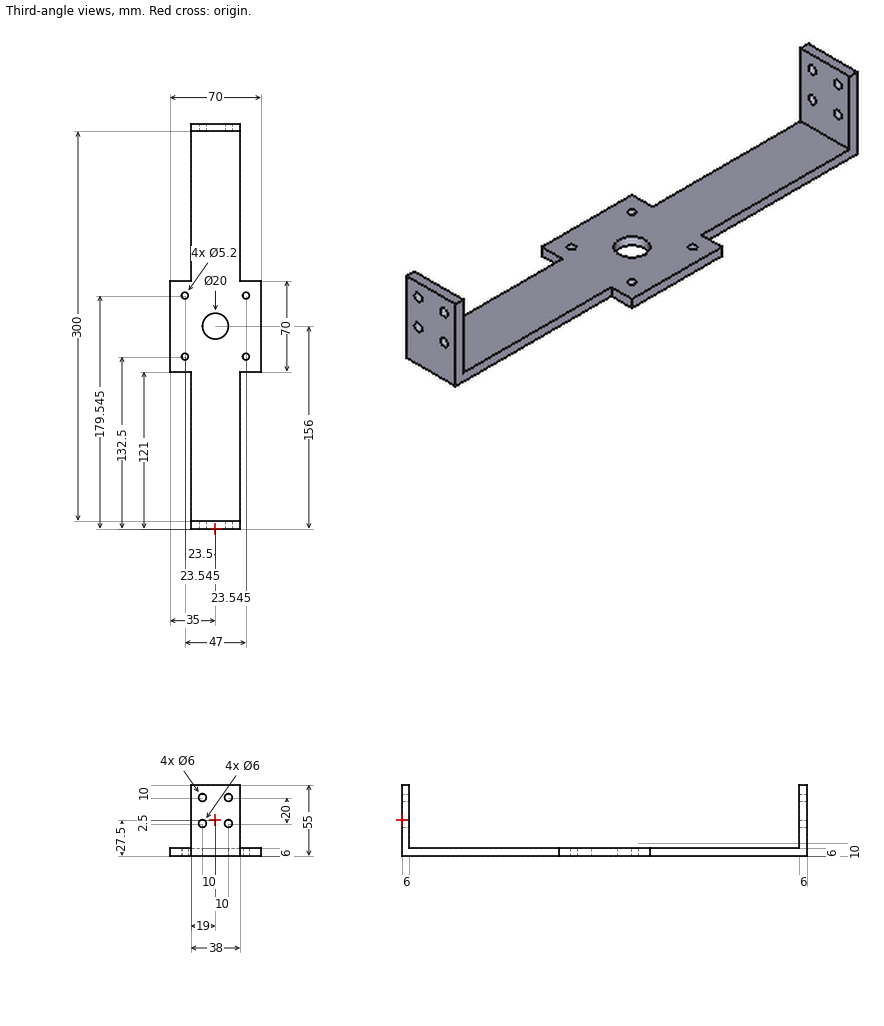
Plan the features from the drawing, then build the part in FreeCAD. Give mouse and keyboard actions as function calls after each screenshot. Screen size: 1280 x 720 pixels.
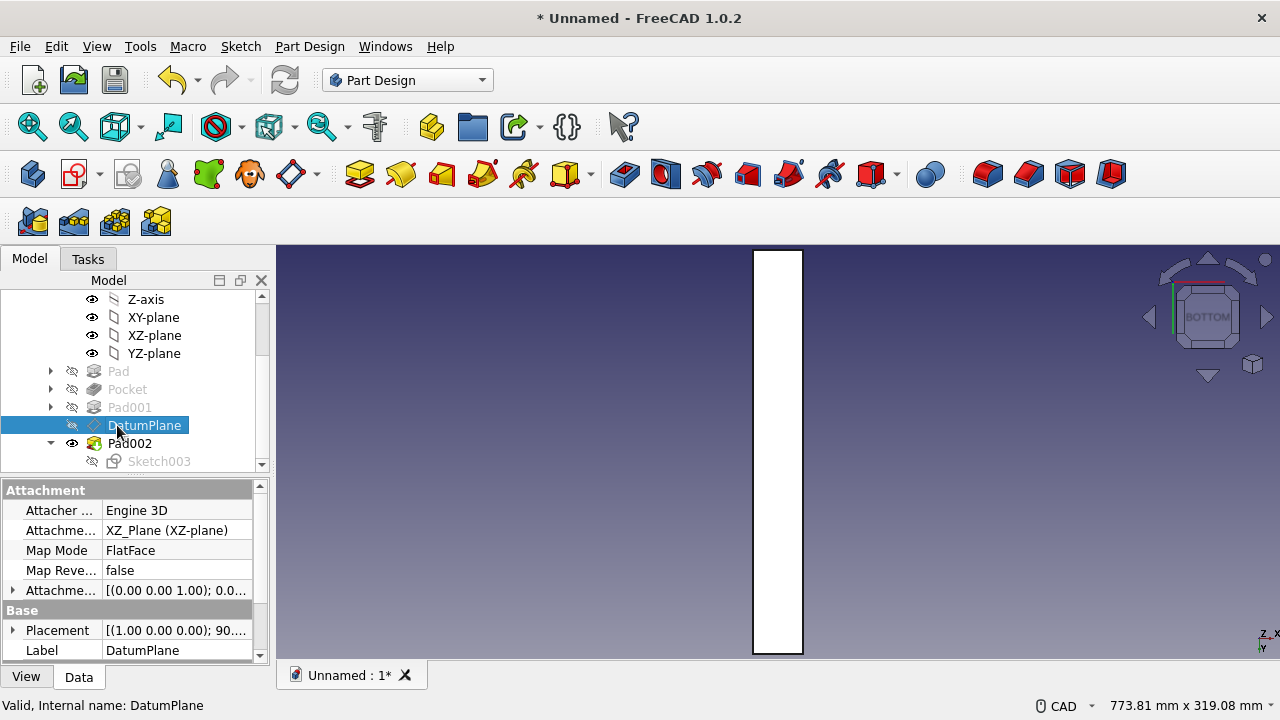
click(778, 624)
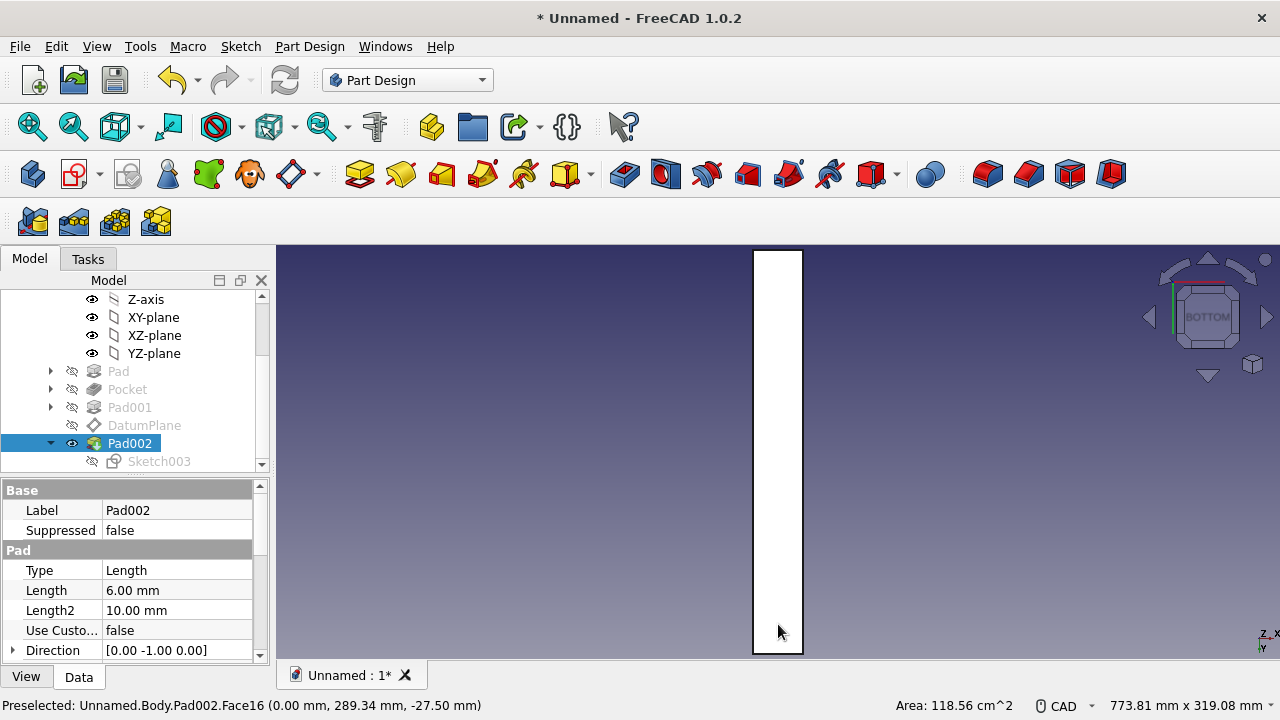
click(74, 174)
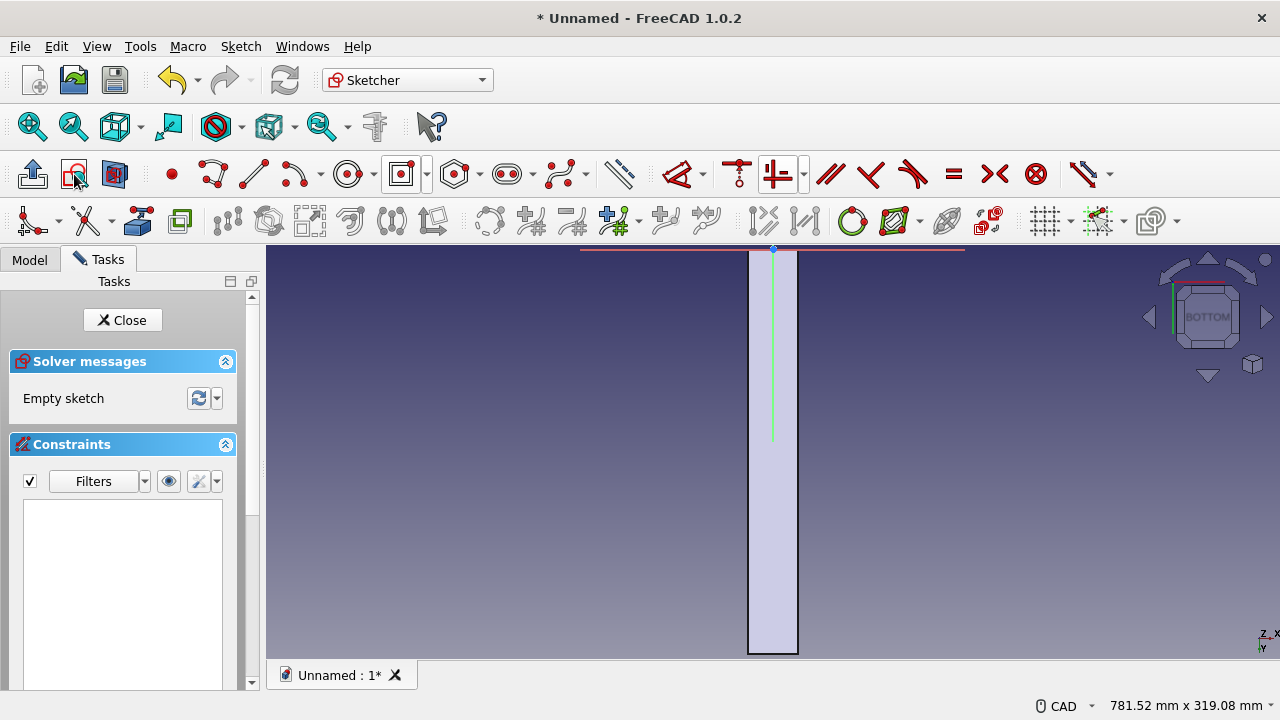
scroll(813, 452, up, 5)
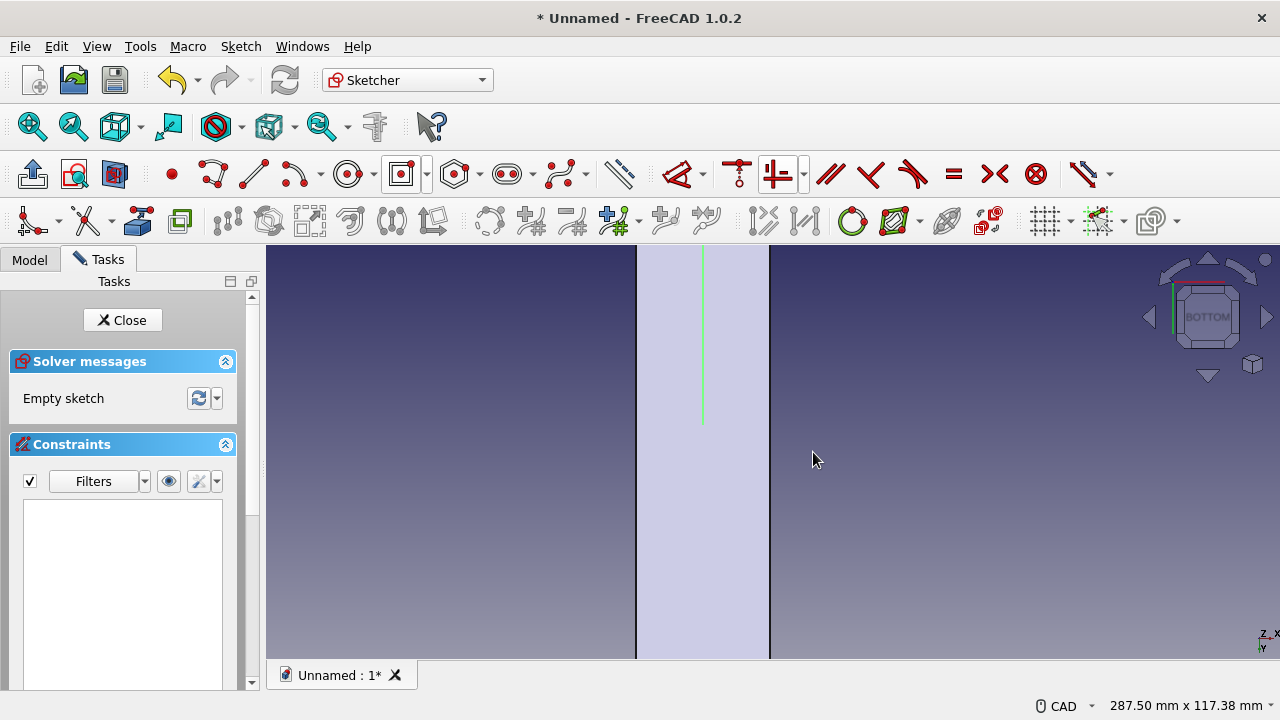
key(g)
key(r)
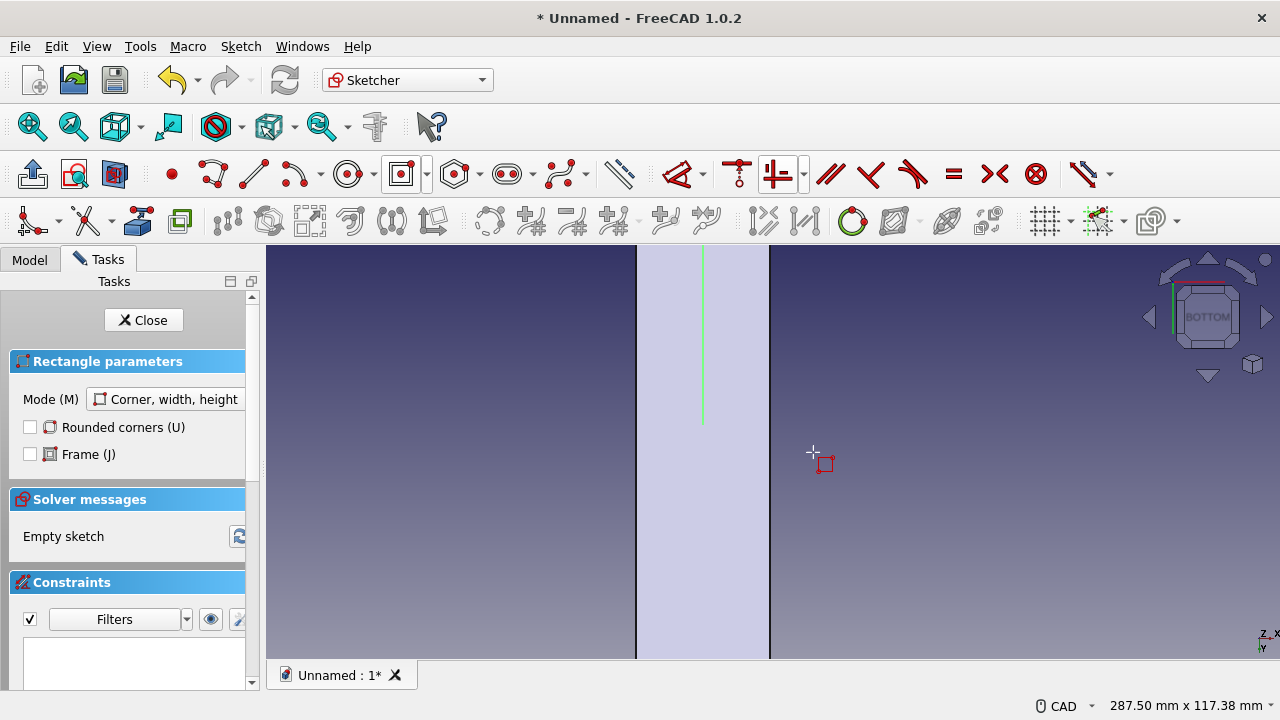
click(580, 328)
move(827, 575)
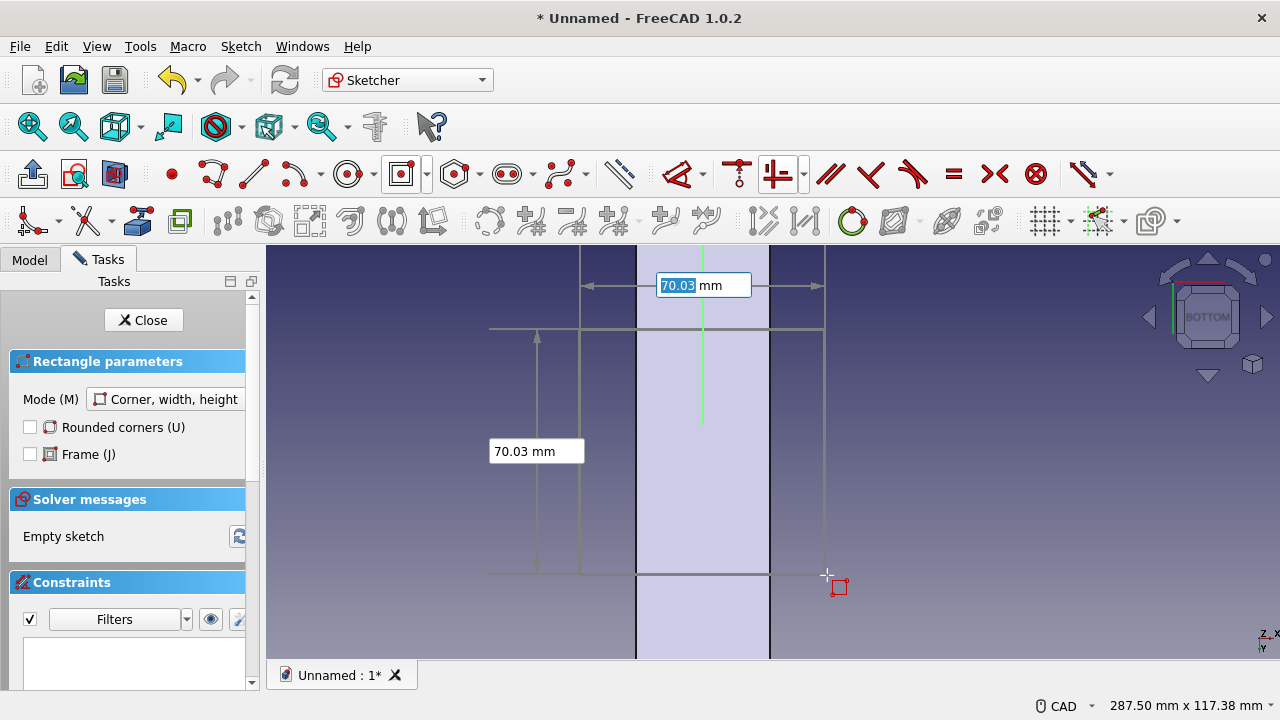
text(70)
key(Tab)
text(70)
key(Return)
key(Escape)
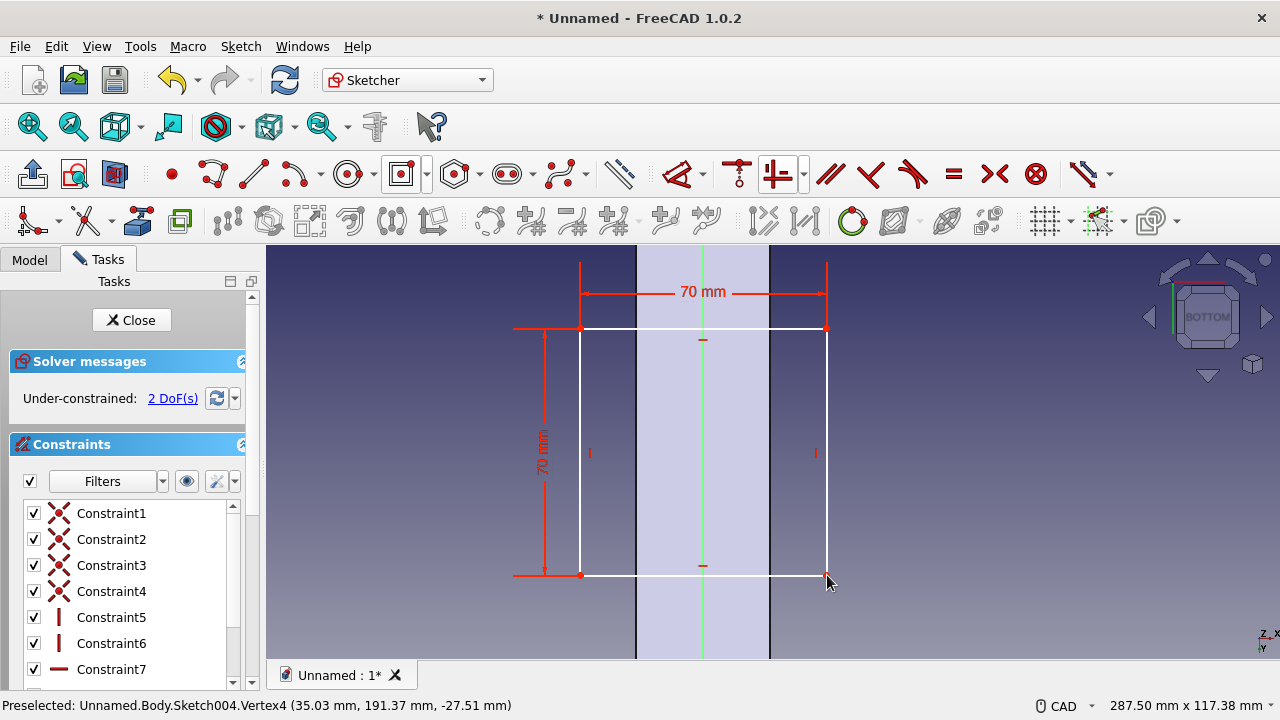
click(676, 174)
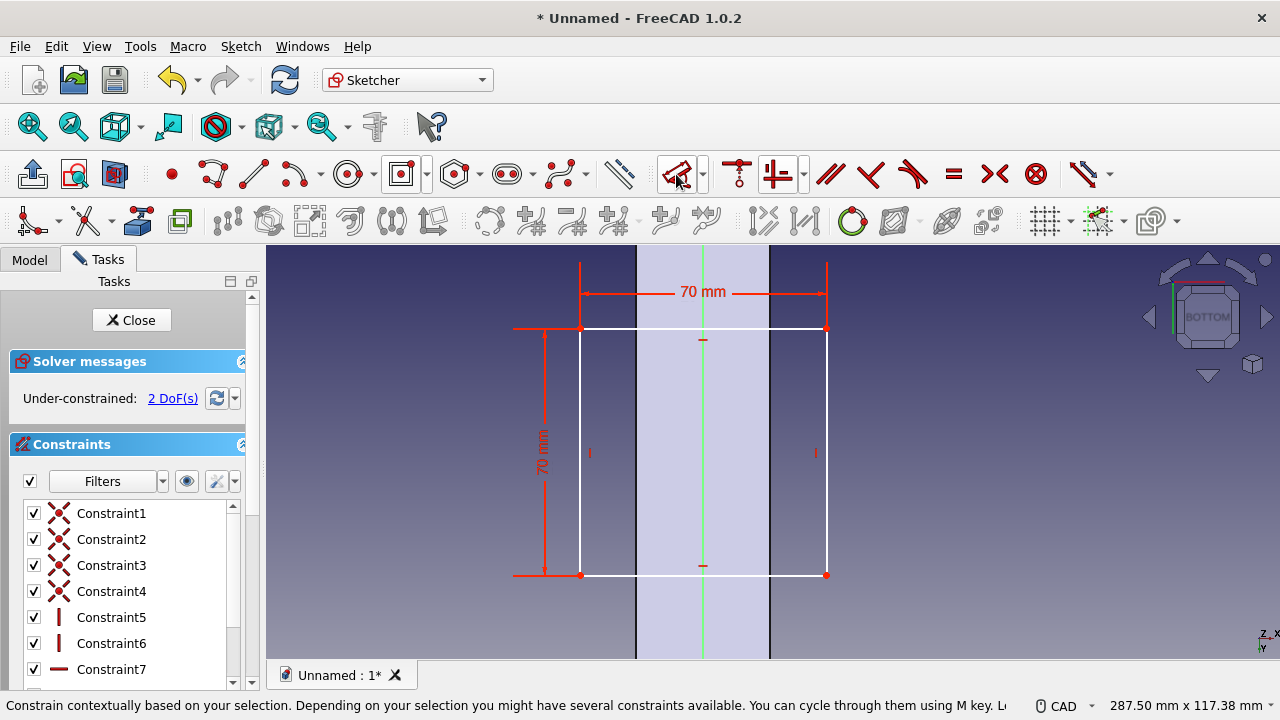
click(580, 329)
click(642, 363)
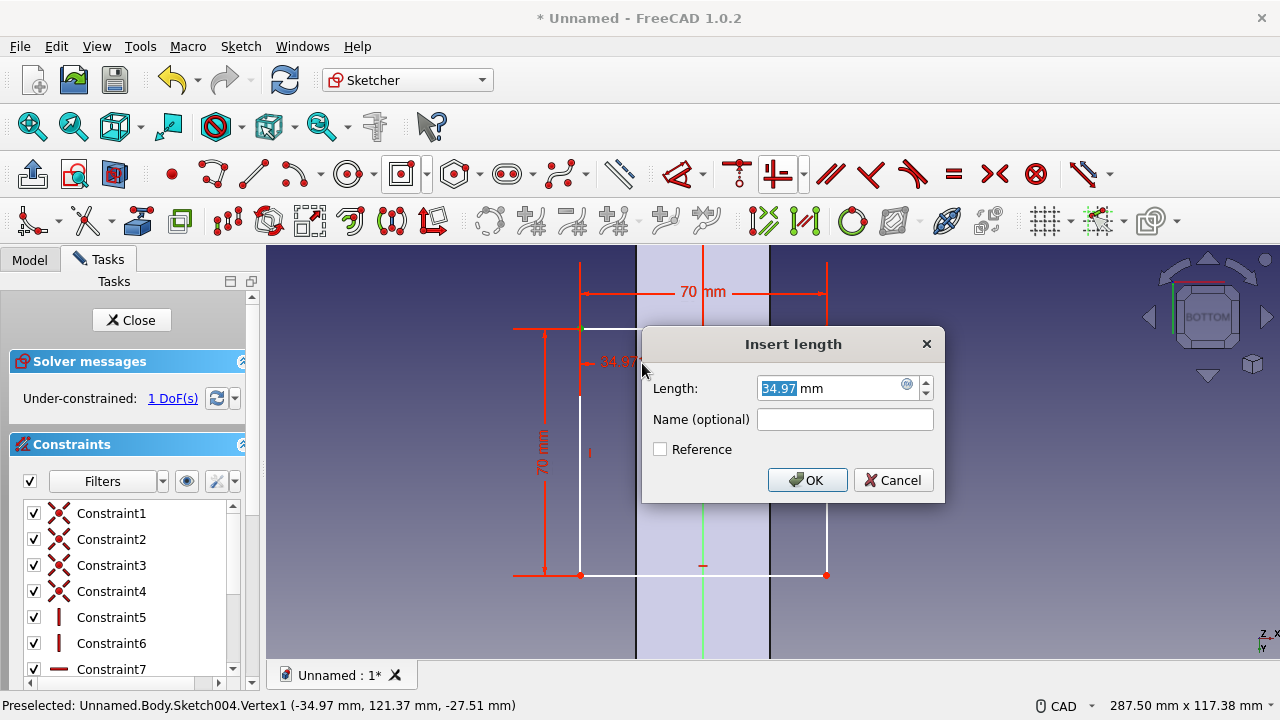
text(35)
key(Return)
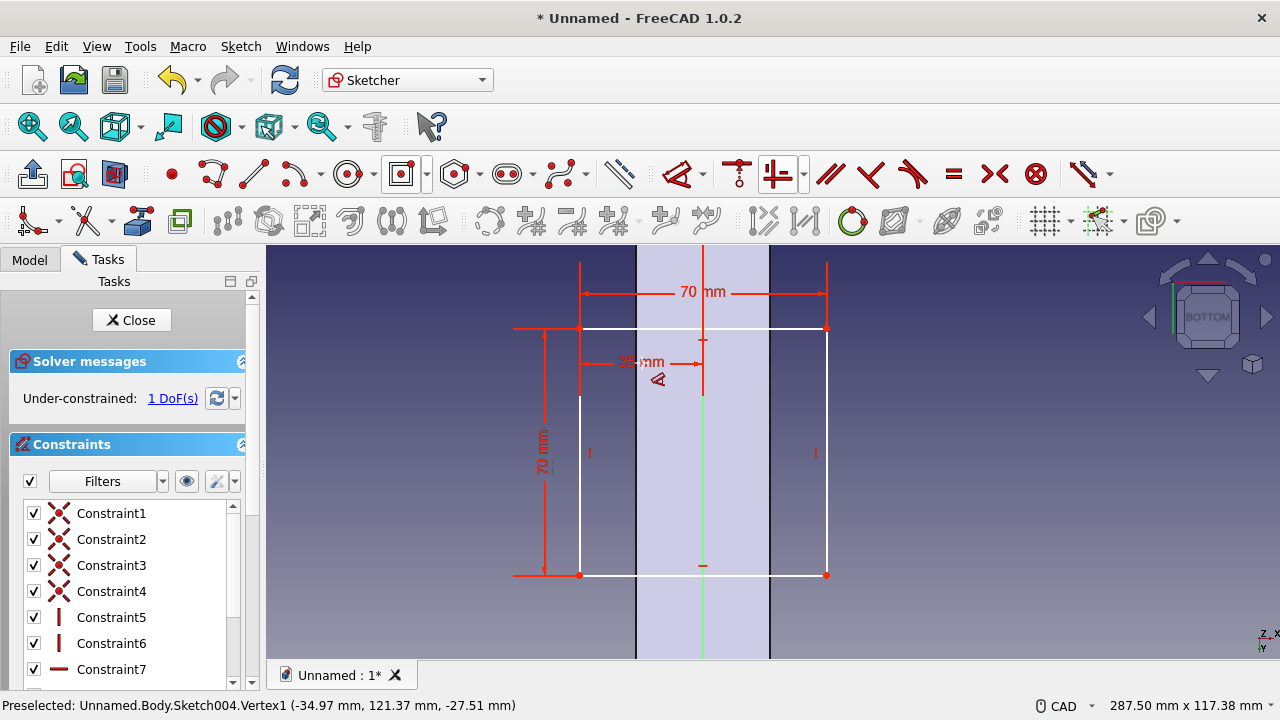
click(580, 329)
click(546, 301)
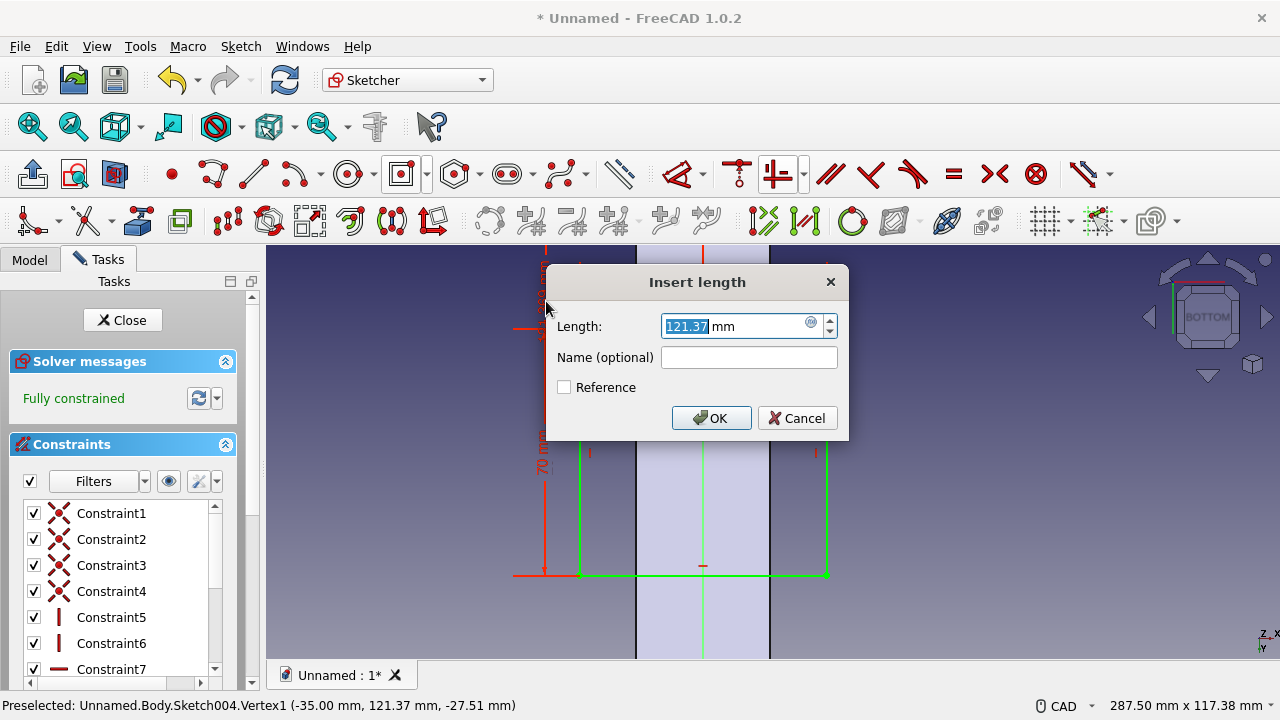
text(121)
key(Return)
key(Escape)